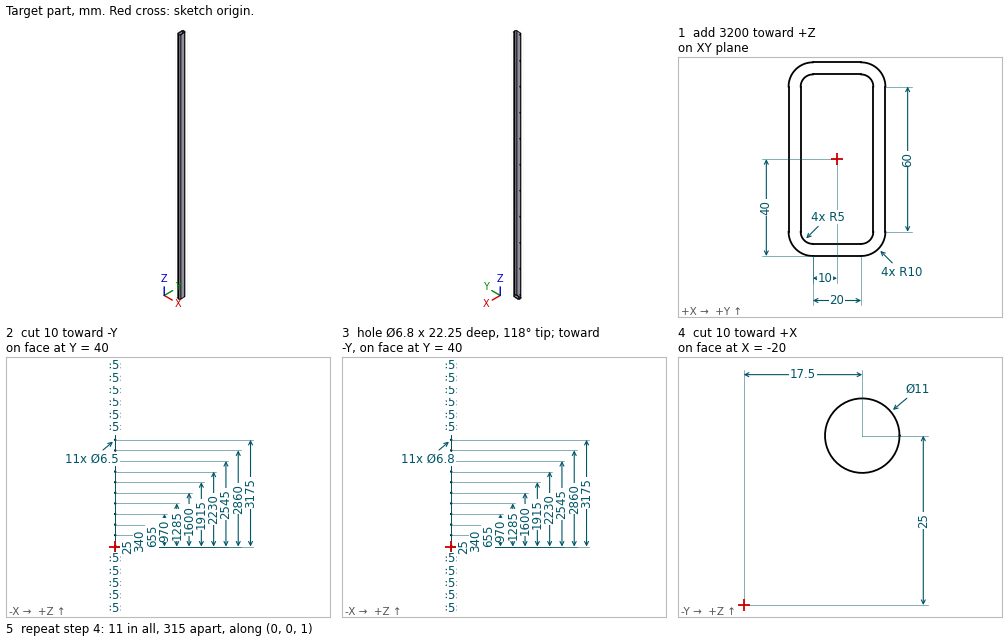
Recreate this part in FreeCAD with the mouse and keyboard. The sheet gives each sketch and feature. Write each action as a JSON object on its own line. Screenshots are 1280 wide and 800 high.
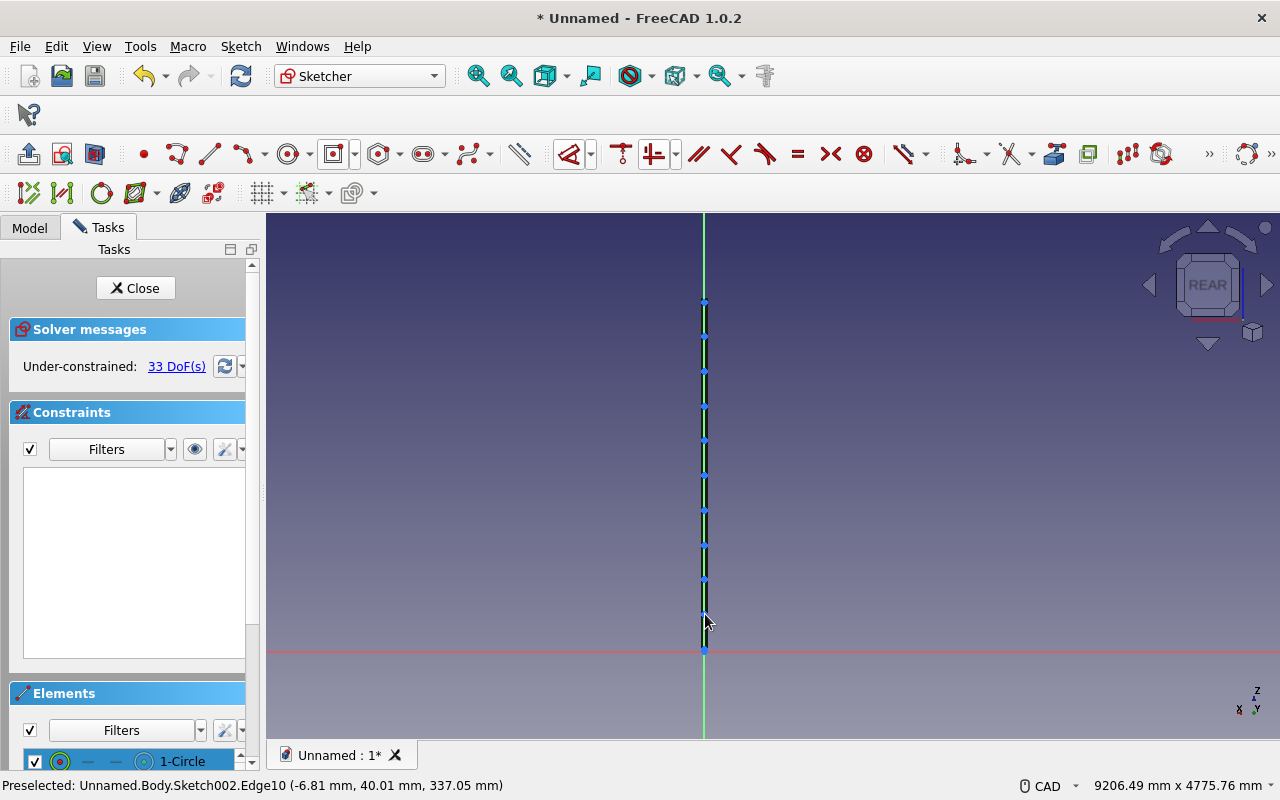
{"action": "scroll", "coordinate": [705, 649], "scroll_direction": "up", "scroll_amount": 14}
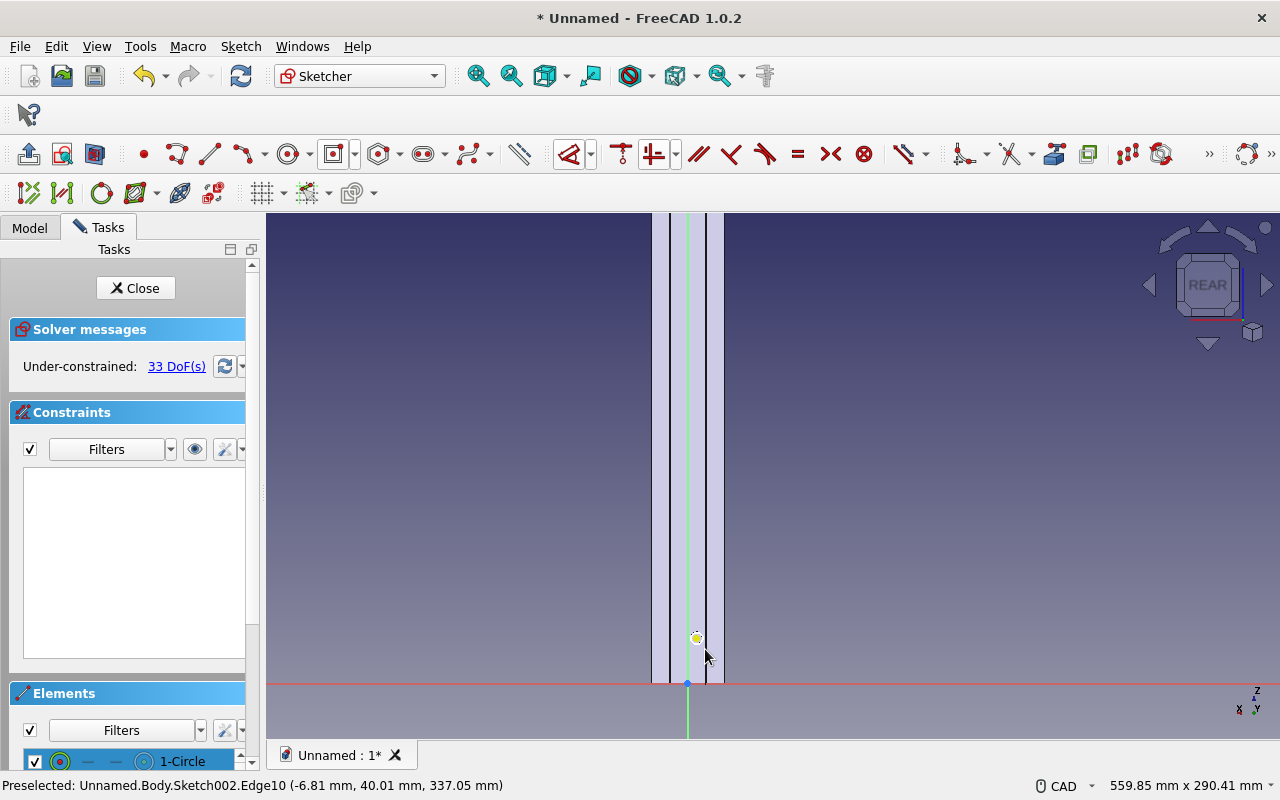
{"action": "left_click", "coordinate": [701, 634]}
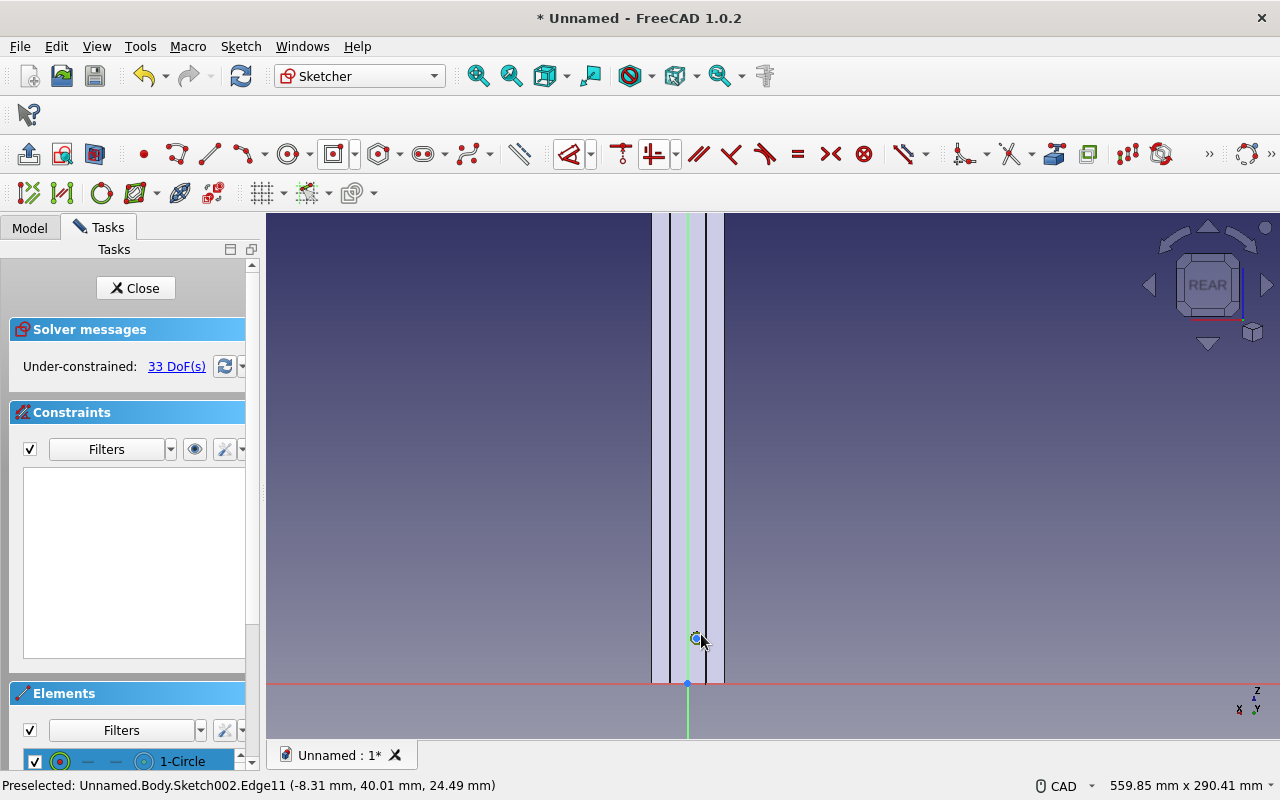
{"action": "left_click", "coordinate": [798, 154]}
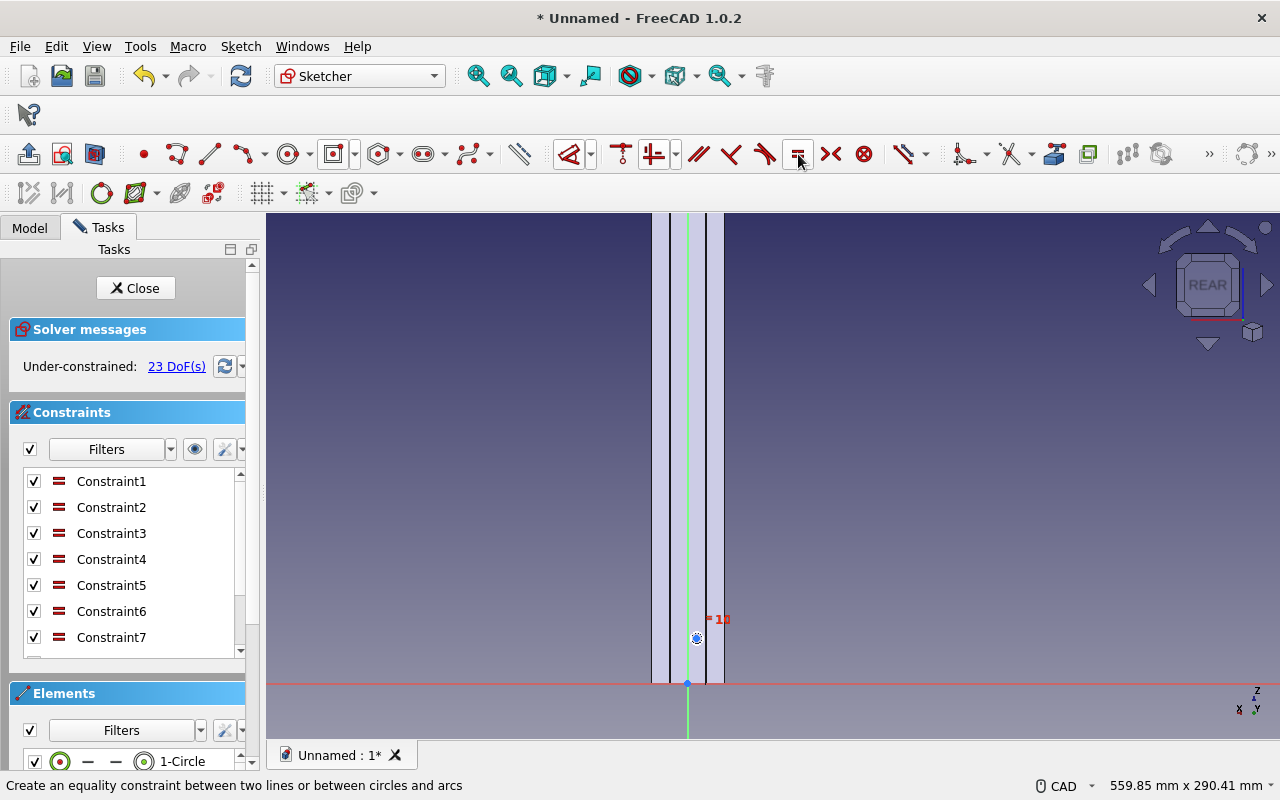
{"action": "scroll", "coordinate": [705, 649], "scroll_direction": "down", "scroll_amount": 14}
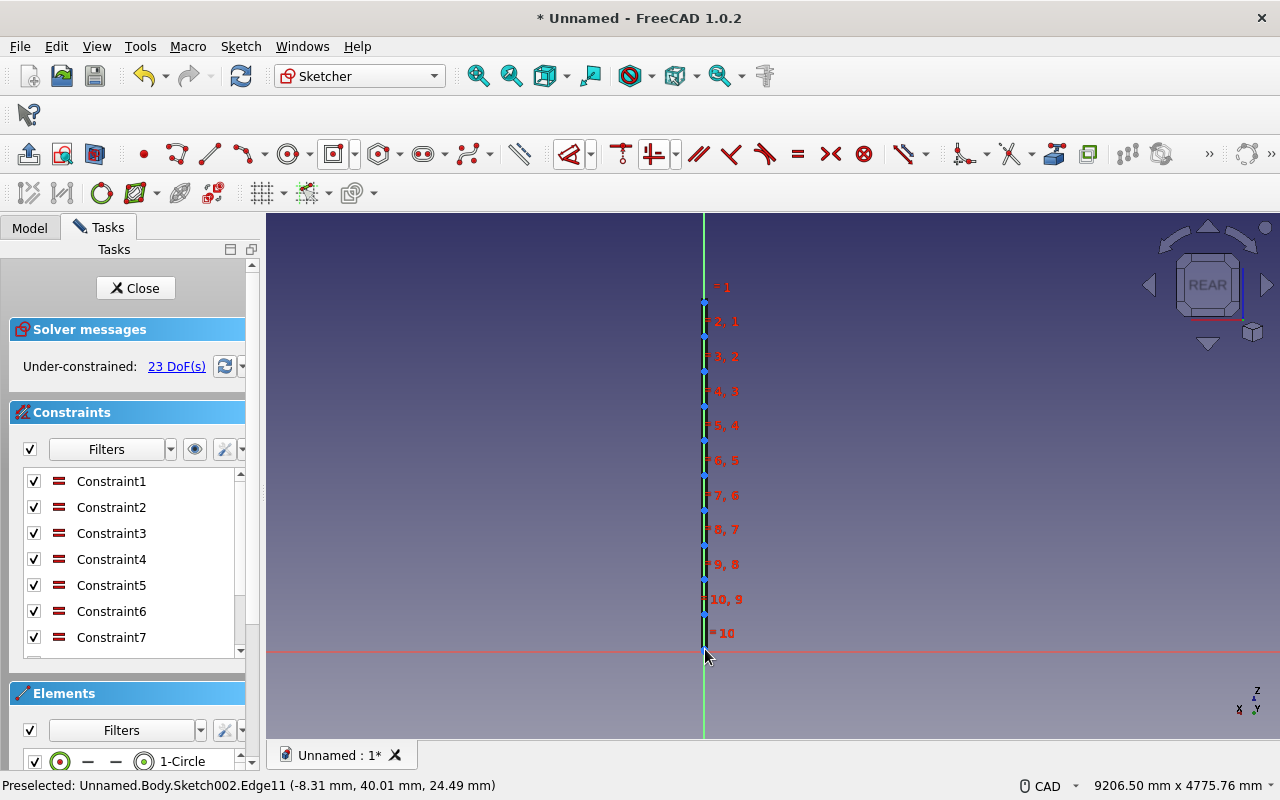
{"action": "scroll", "coordinate": [705, 302], "scroll_direction": "up", "scroll_amount": 20}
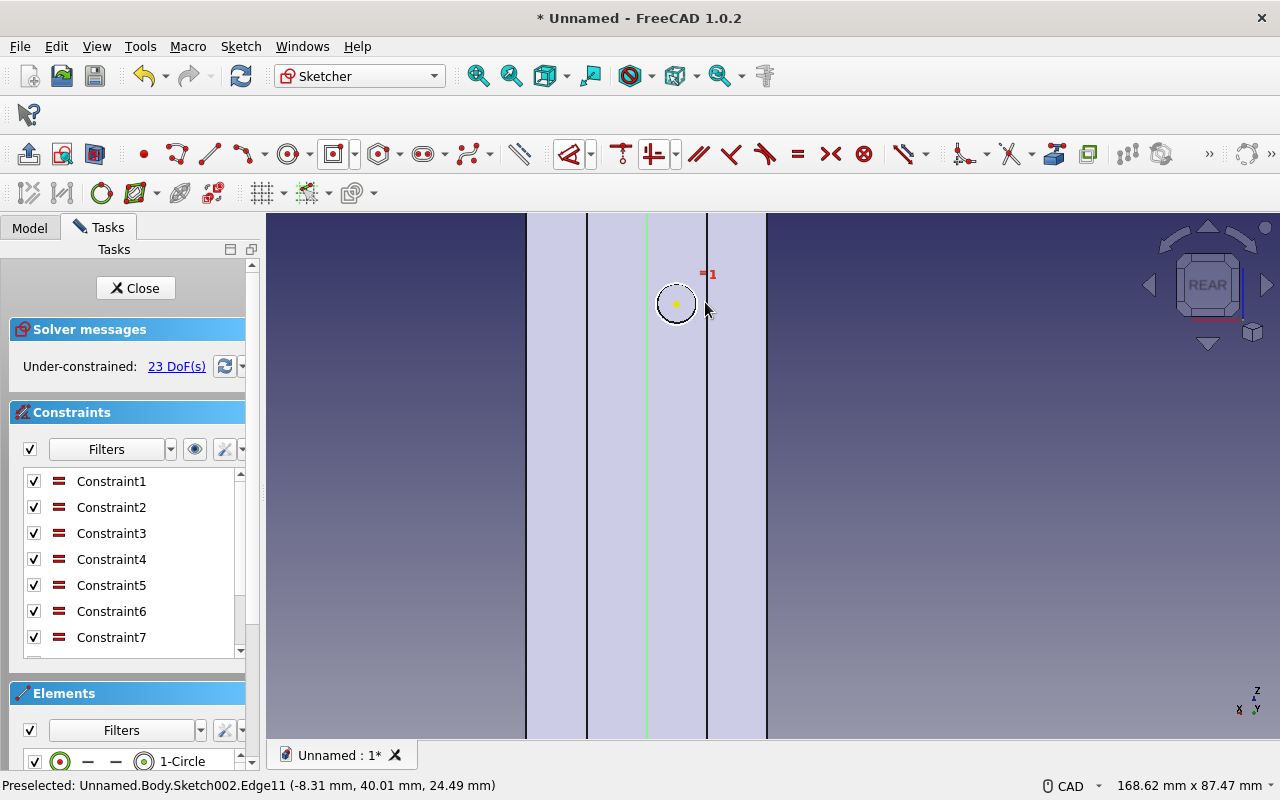
{"action": "left_click", "coordinate": [677, 283]}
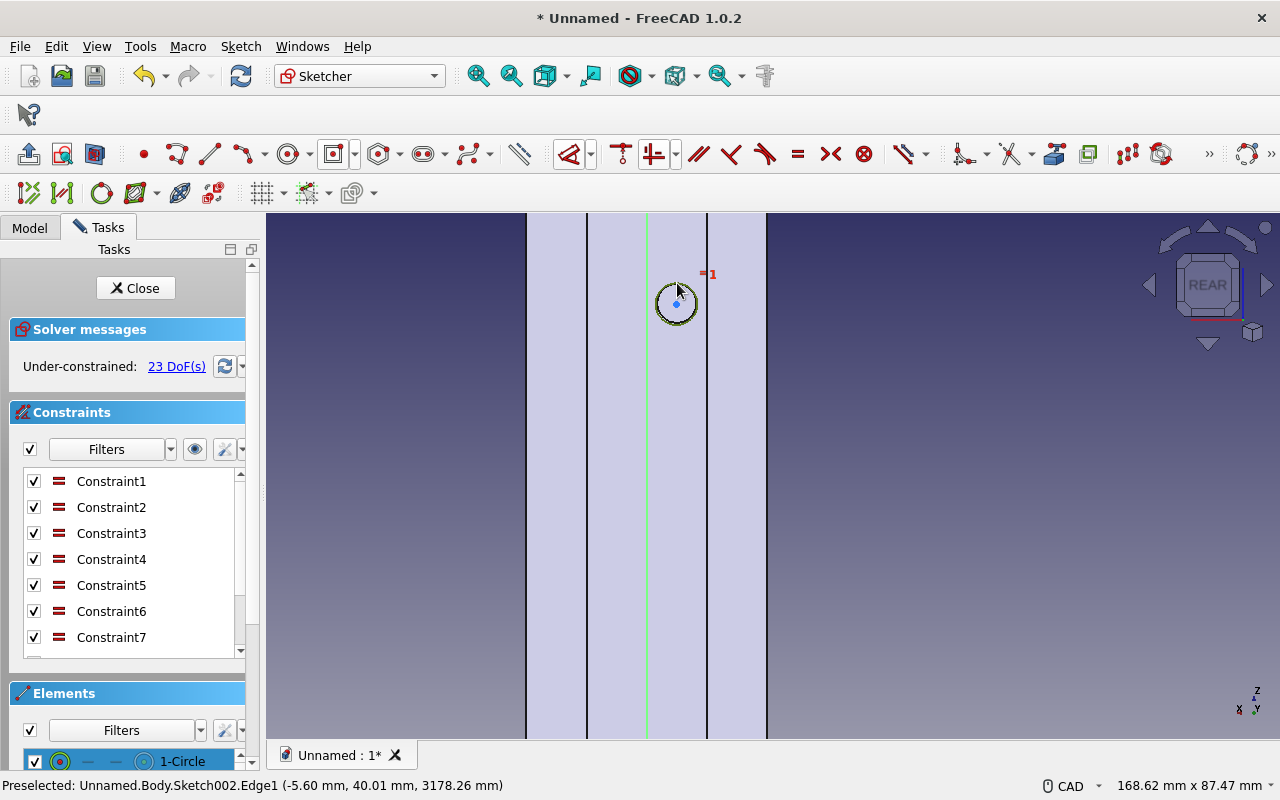
{"action": "key", "text": "k o"}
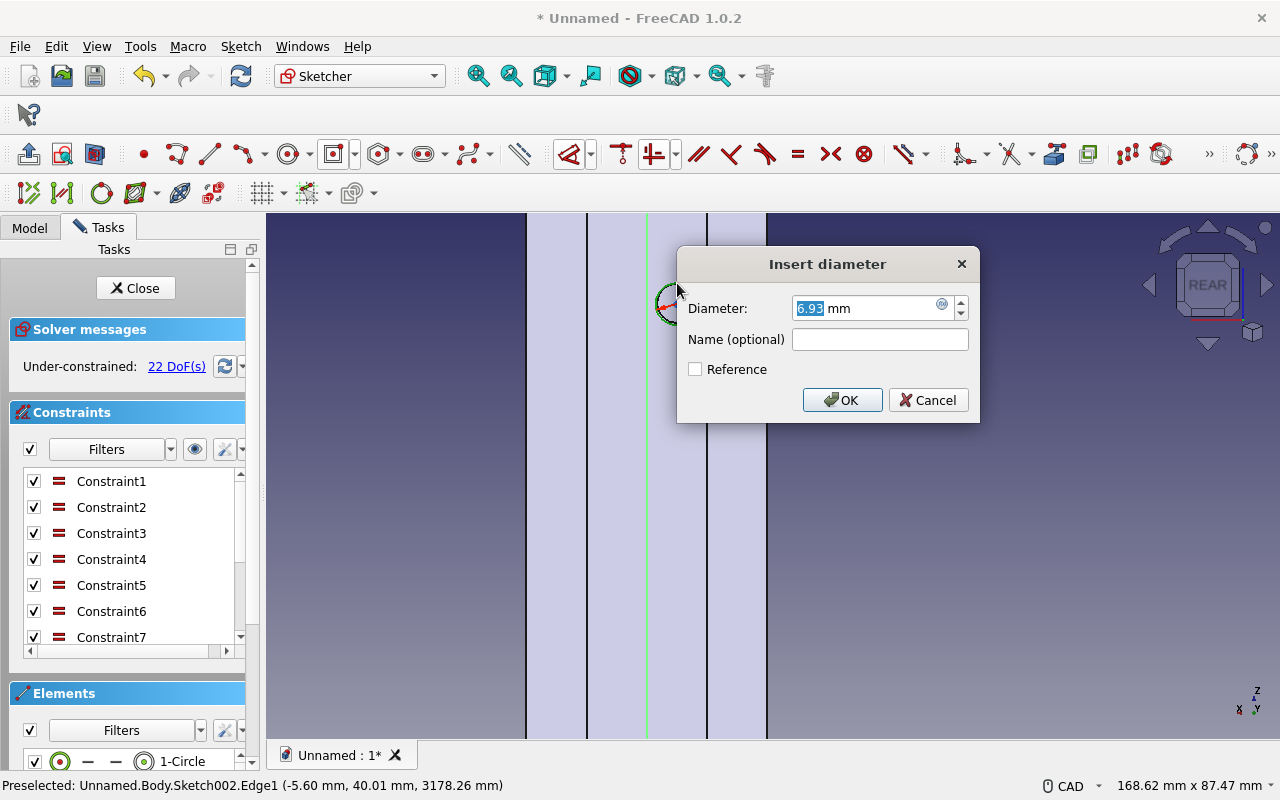
{"action": "type", "text": "6.8"}
{"action": "key", "text": "Return"}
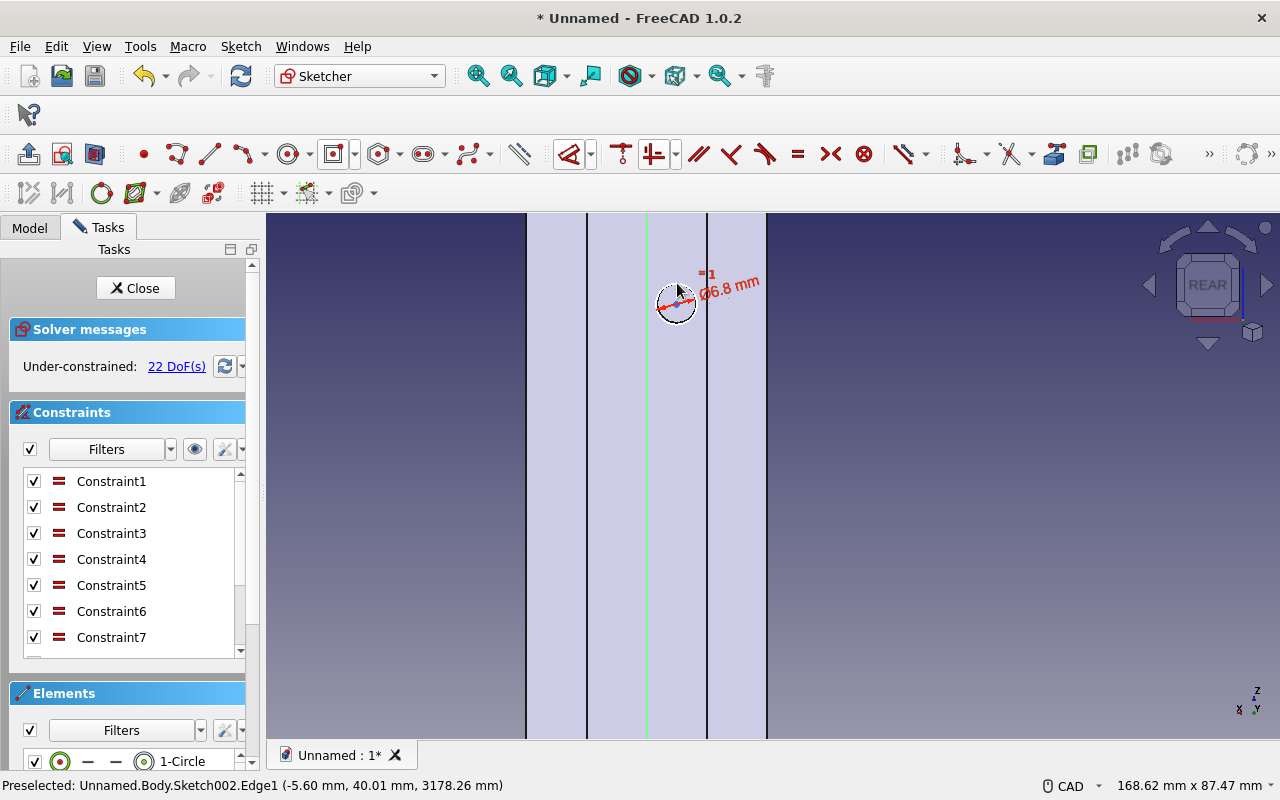
{"action": "scroll", "coordinate": [676, 304], "scroll_direction": "up", "scroll_amount": 2}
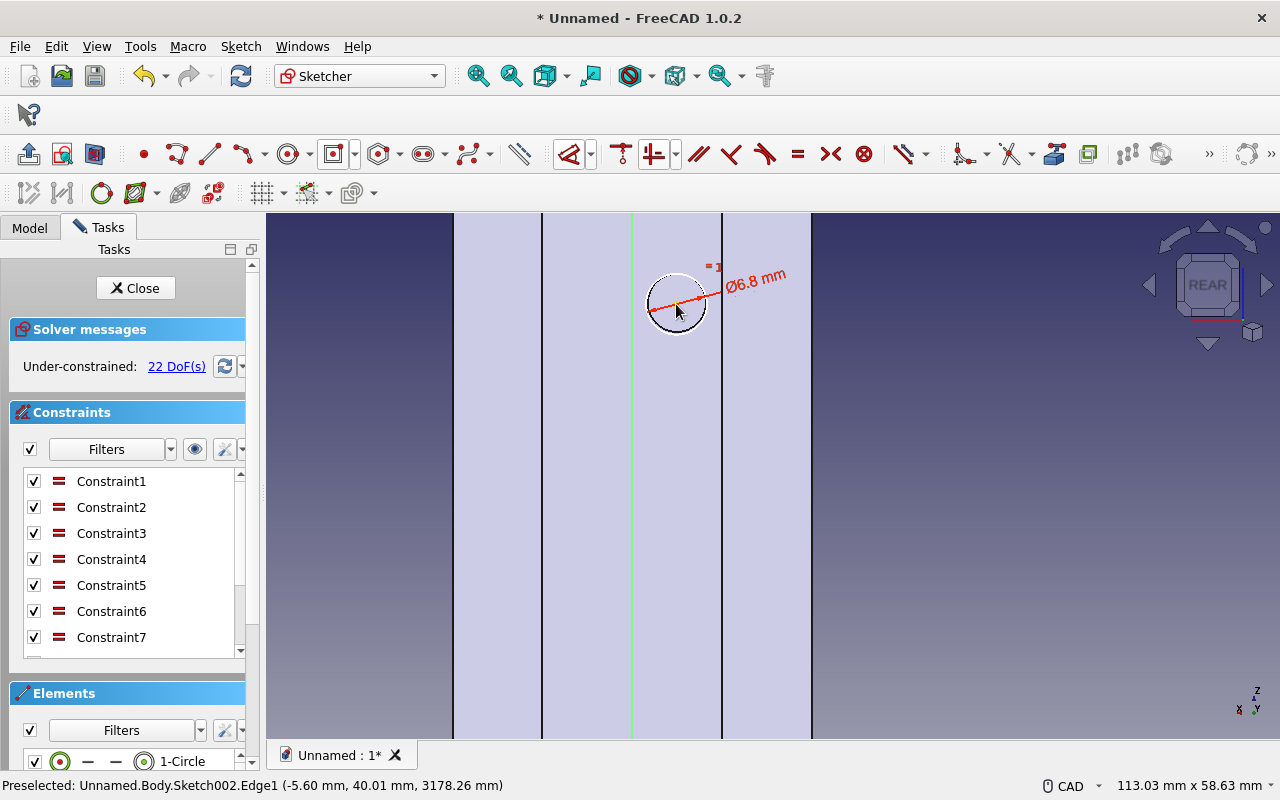
{"action": "left_click", "coordinate": [677, 304]}